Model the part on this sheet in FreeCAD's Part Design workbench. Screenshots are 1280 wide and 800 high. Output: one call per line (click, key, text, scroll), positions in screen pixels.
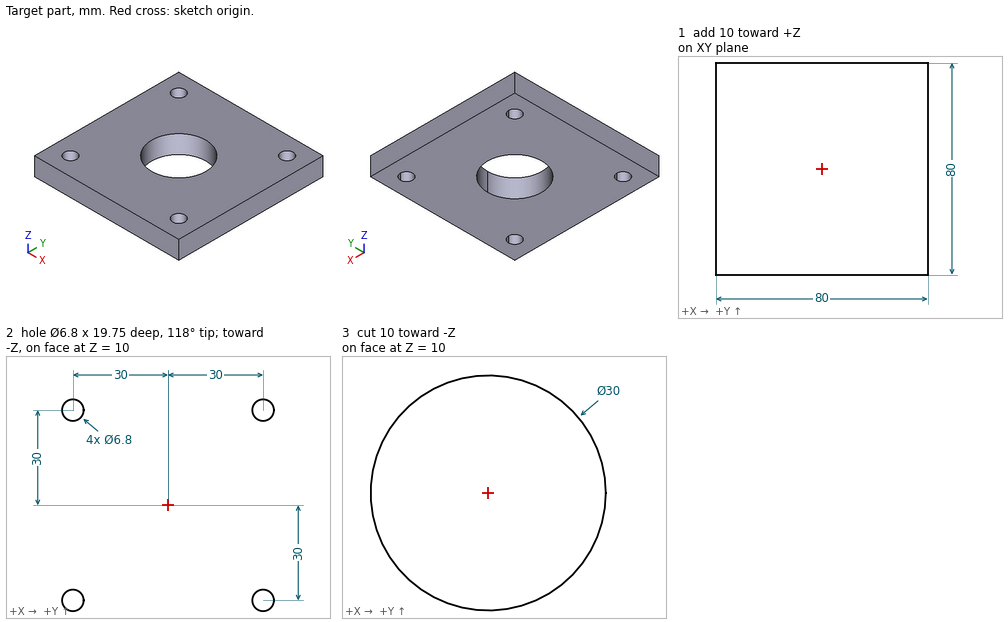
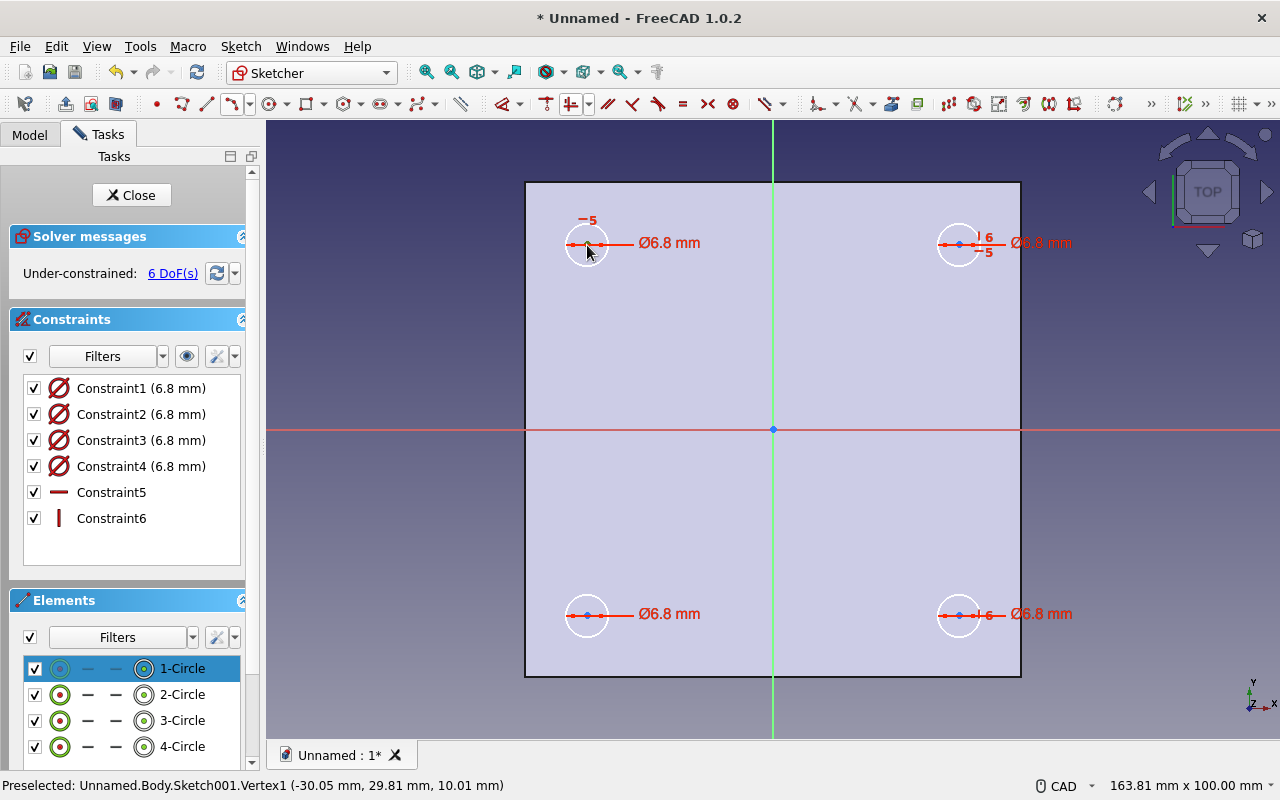
click(587, 616)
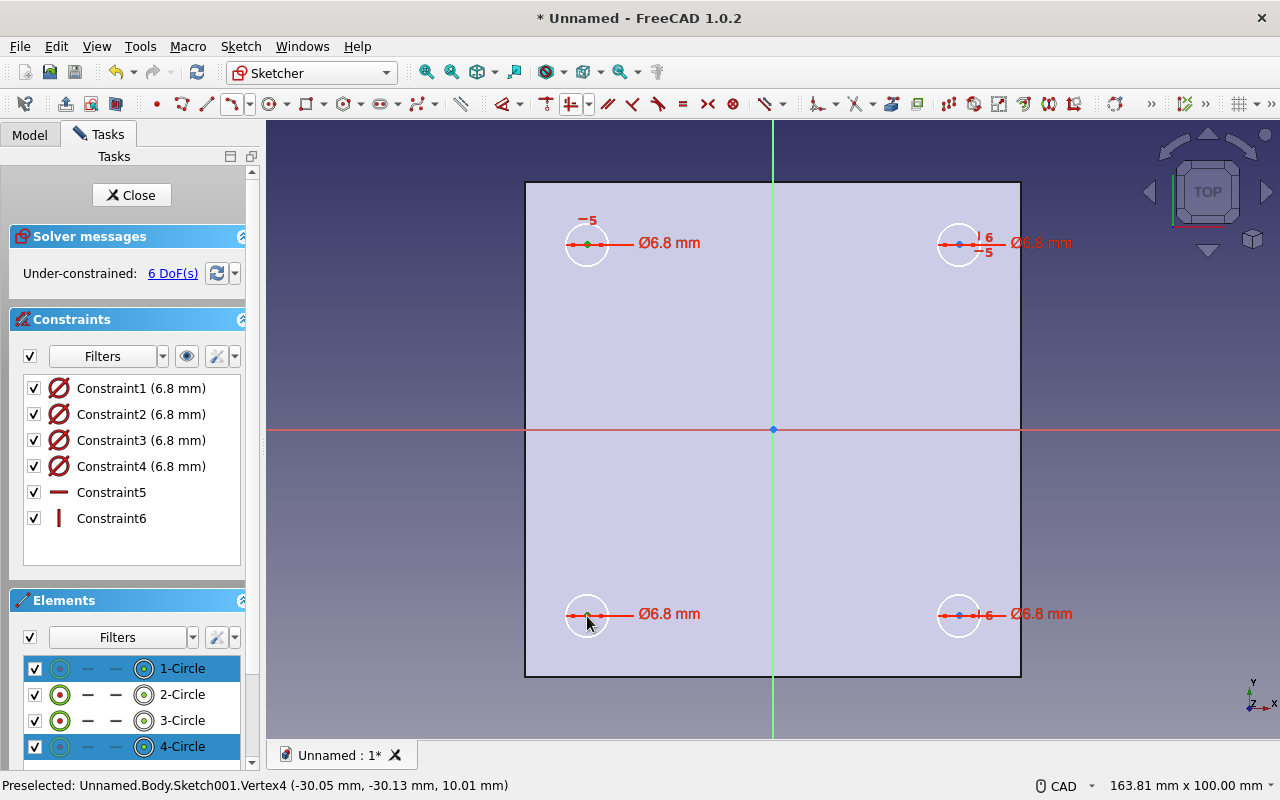
key(v)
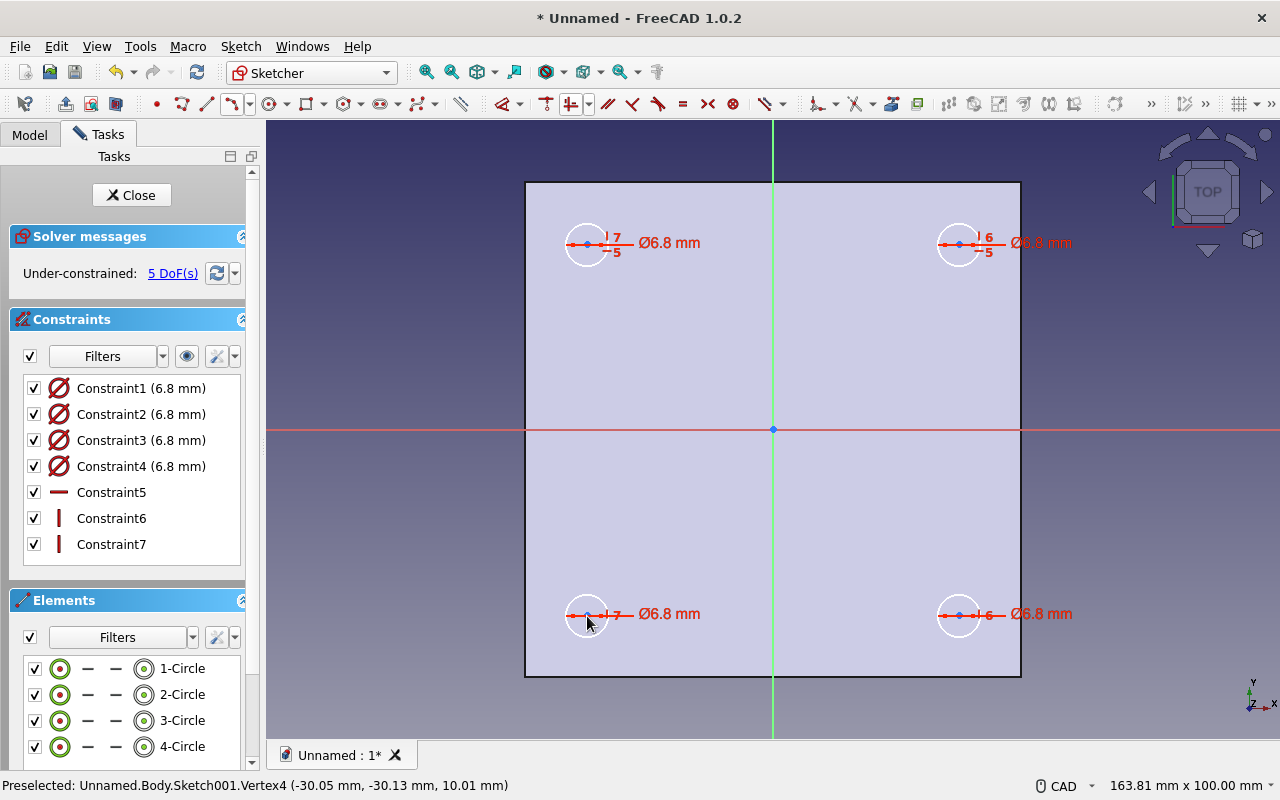
click(959, 616)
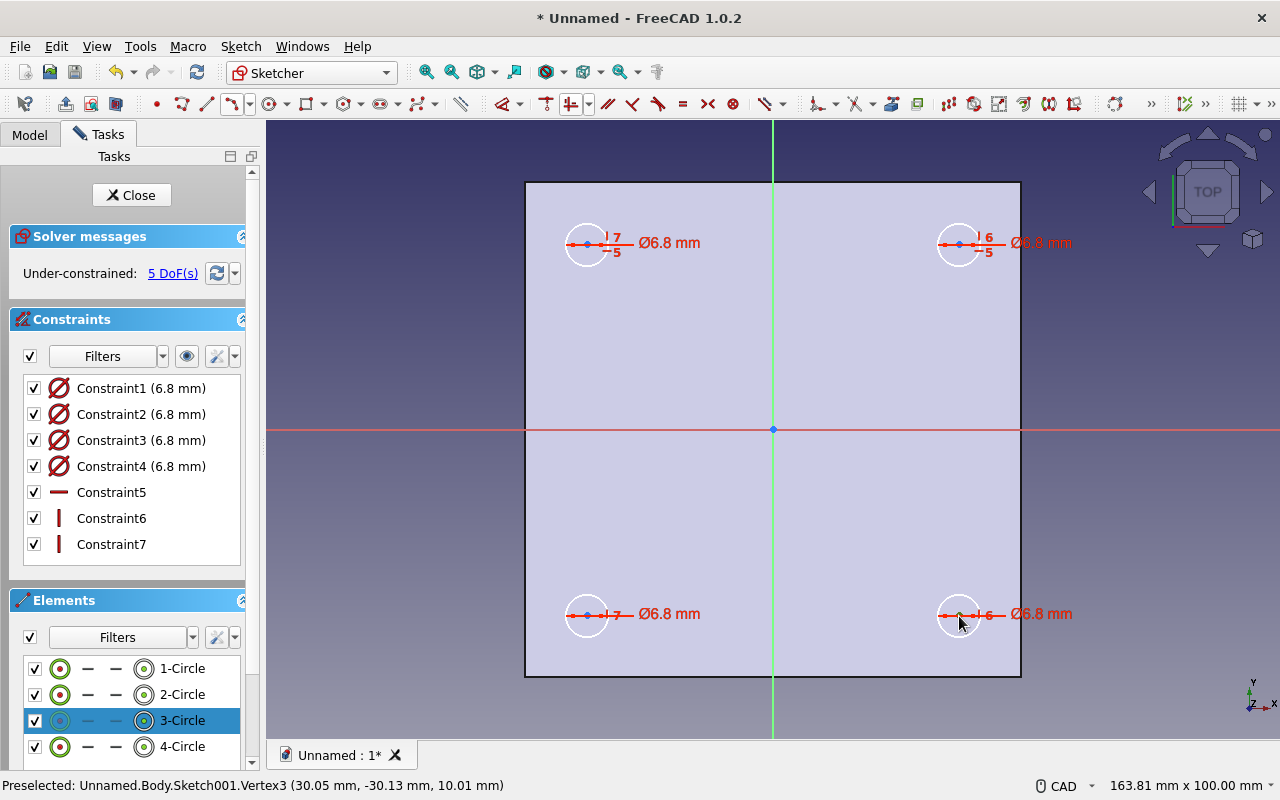
click(587, 616)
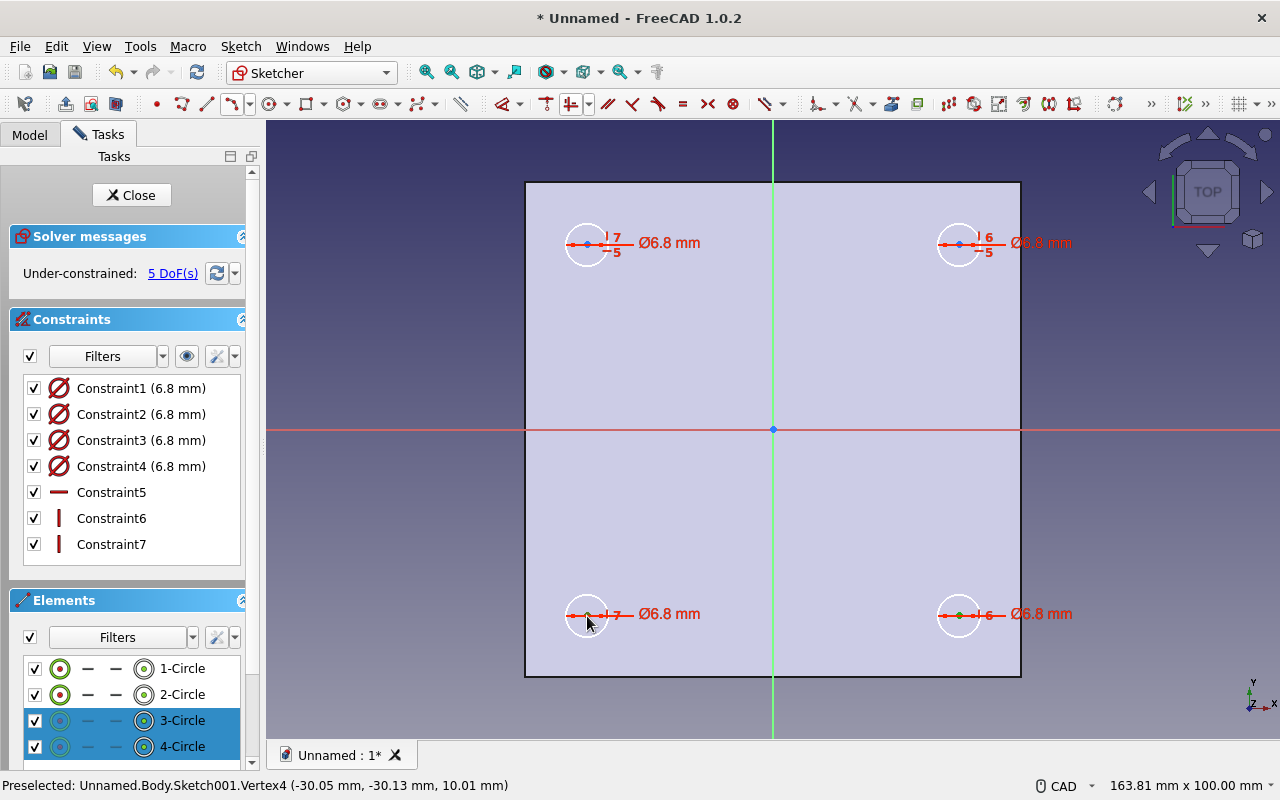
key(h)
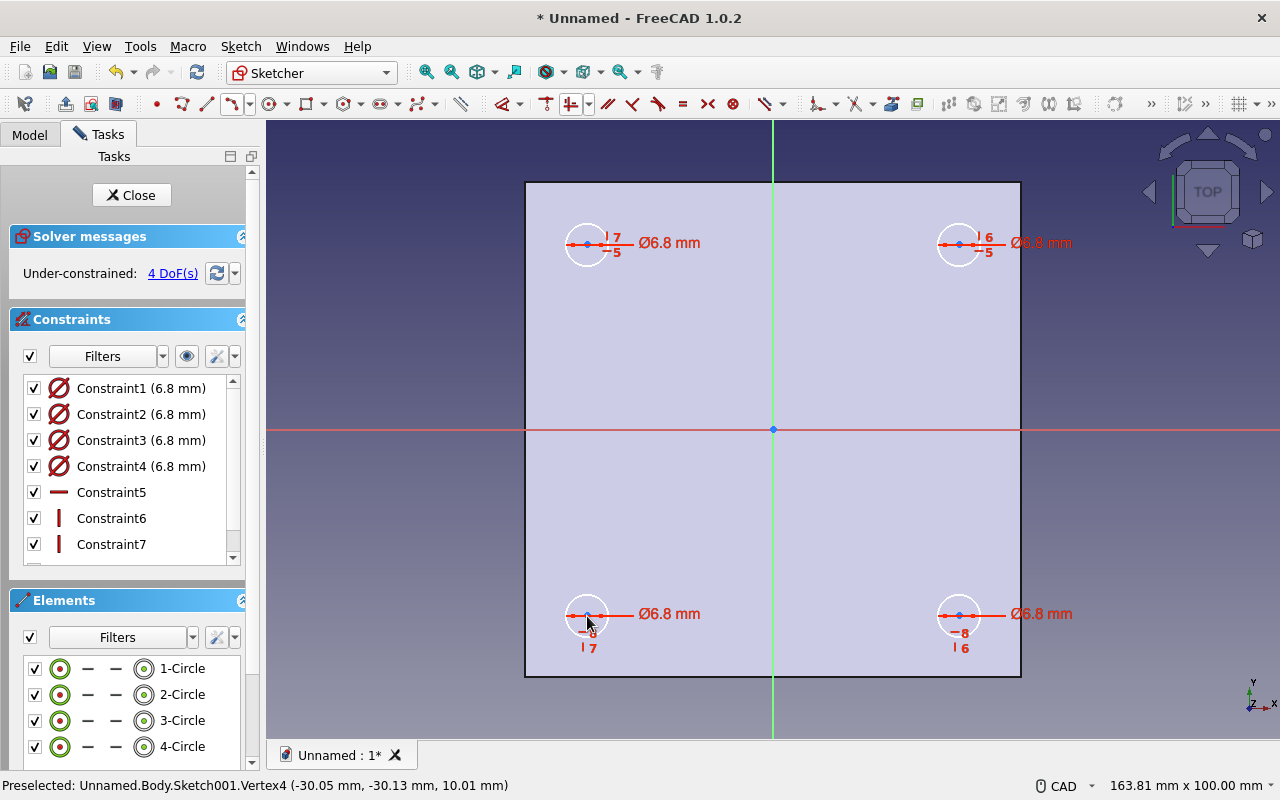
key(d)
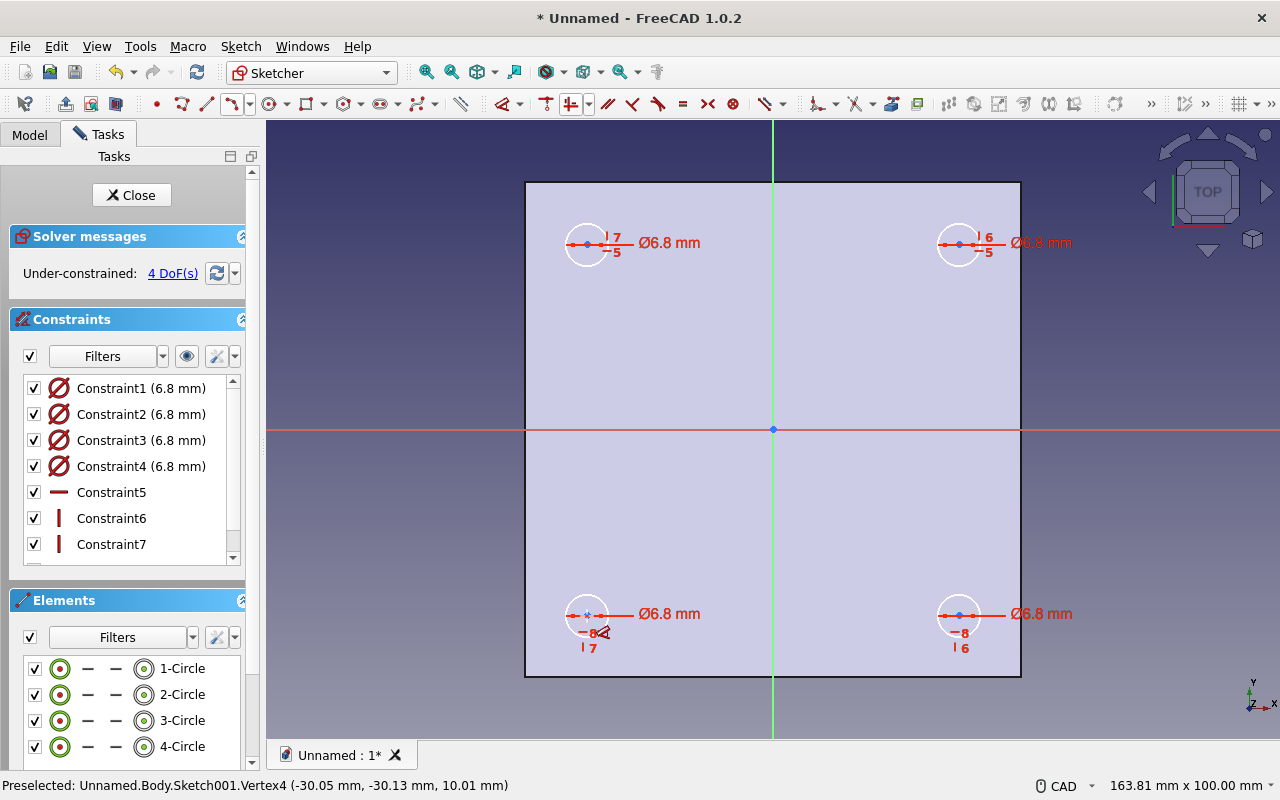
click(587, 245)
click(680, 211)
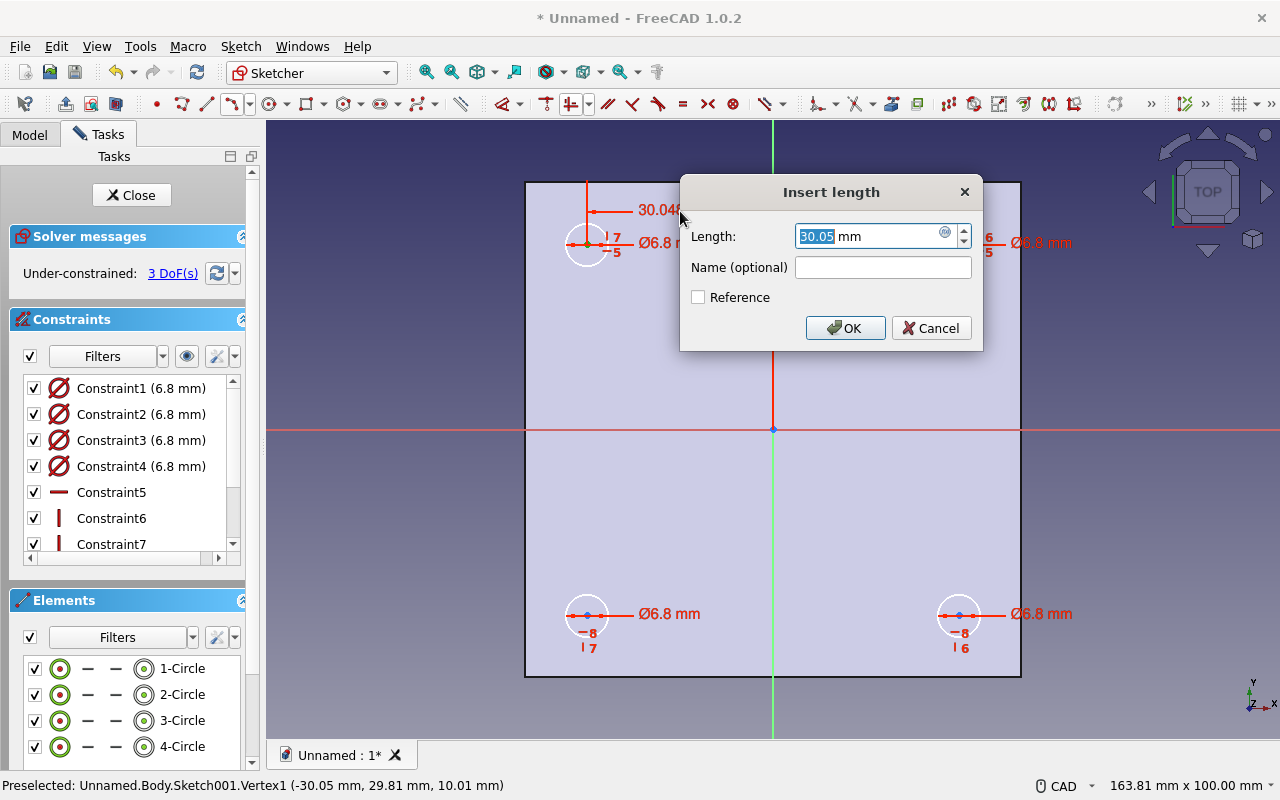
text(30)
key(Return)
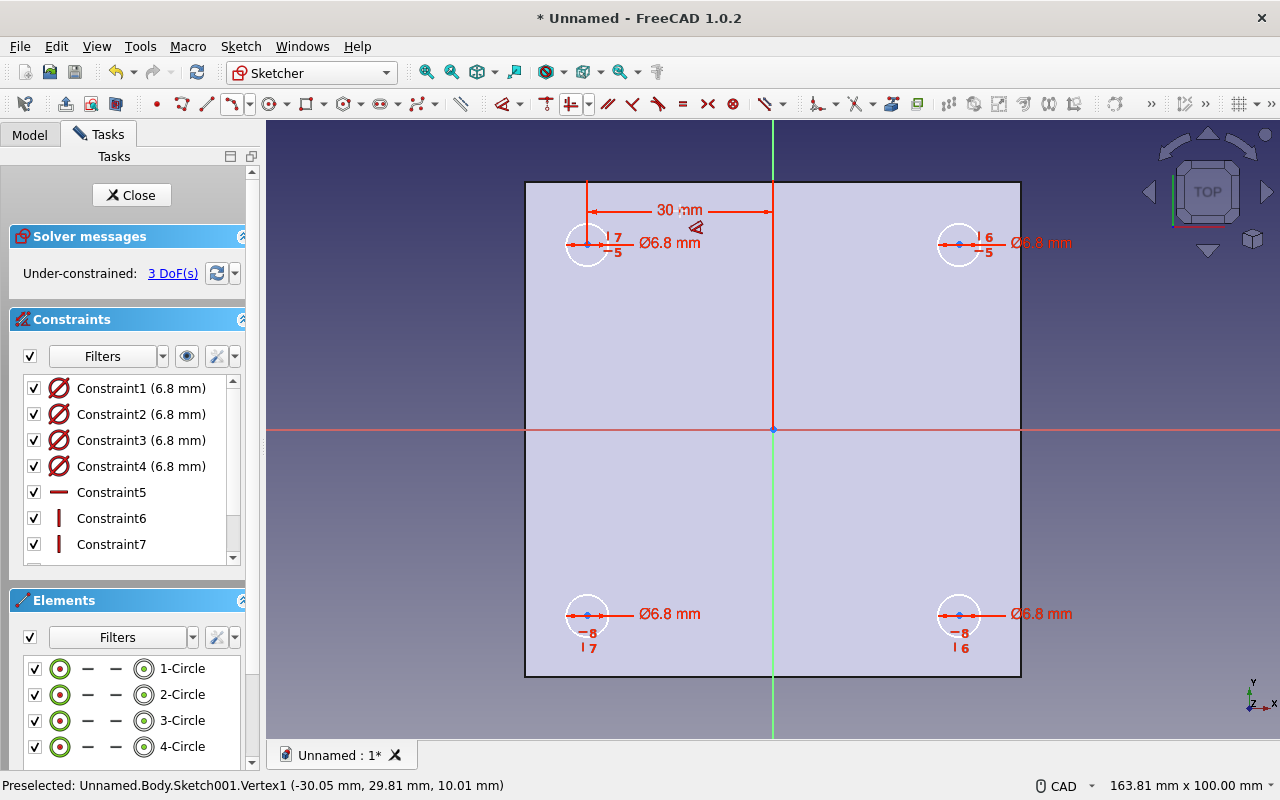
click(587, 245)
click(553, 337)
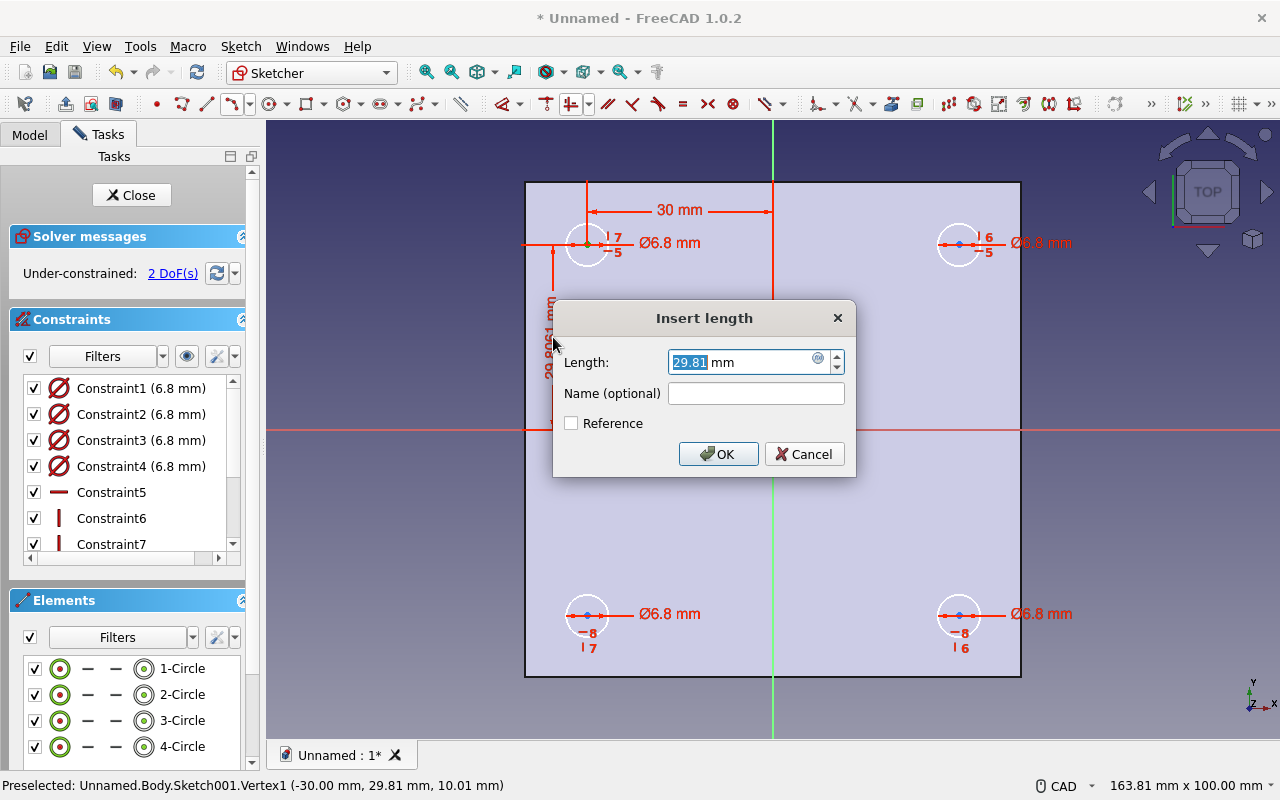
text(30)
key(Return)